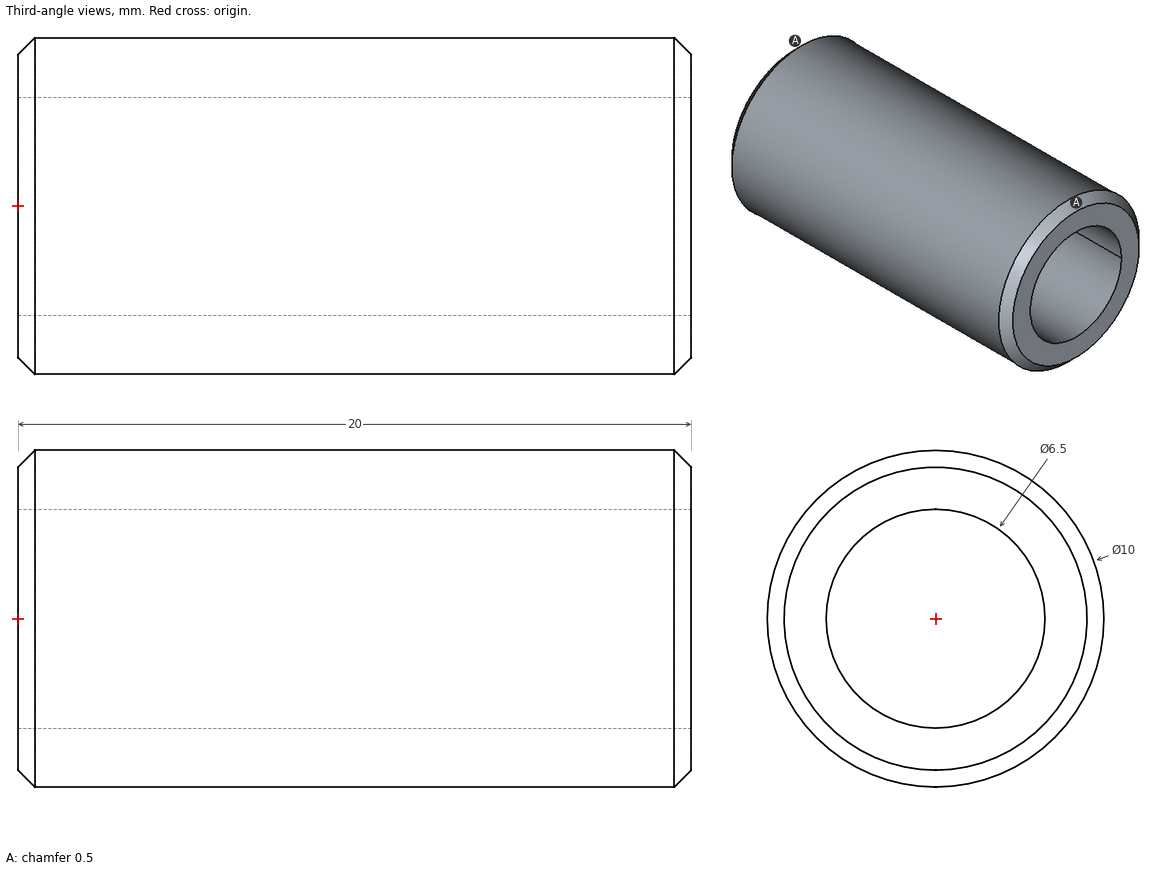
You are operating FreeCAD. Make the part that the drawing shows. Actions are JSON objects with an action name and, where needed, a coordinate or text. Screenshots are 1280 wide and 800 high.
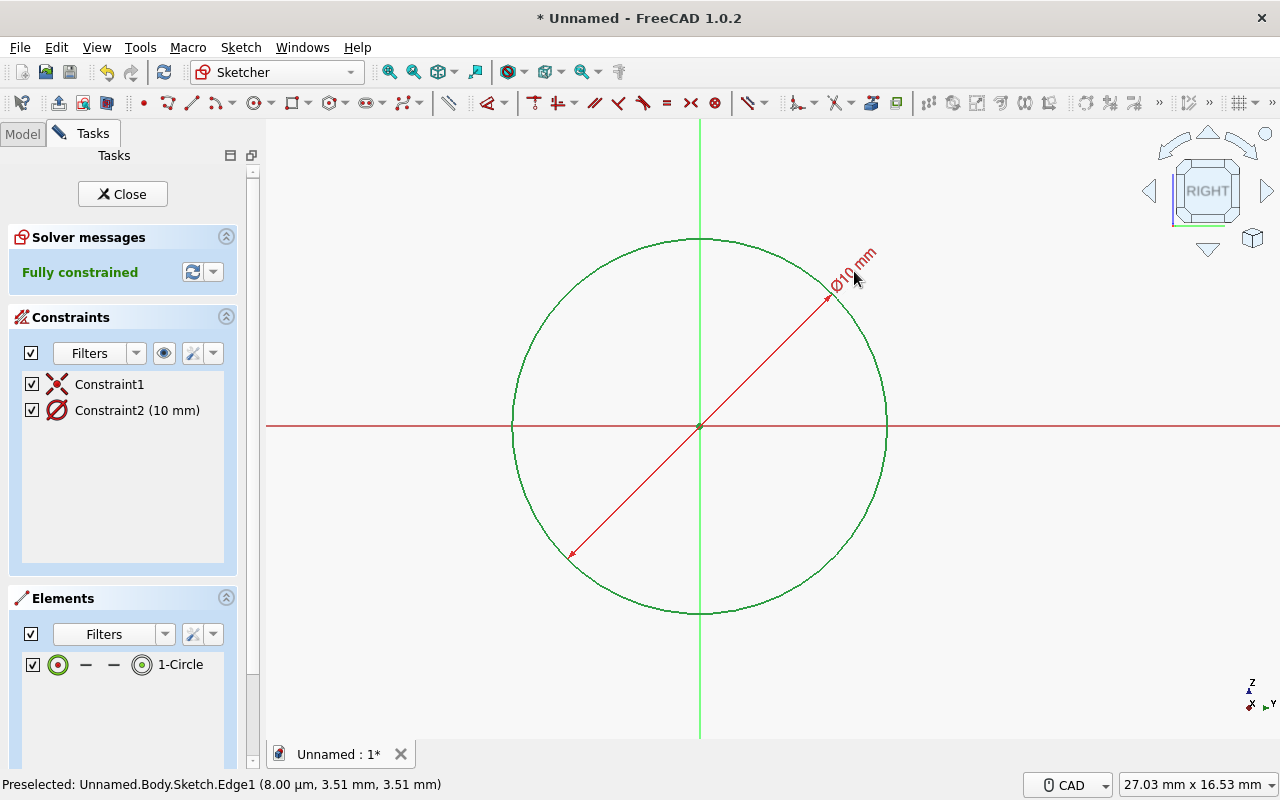
{"action": "left_click", "coordinate": [123, 194]}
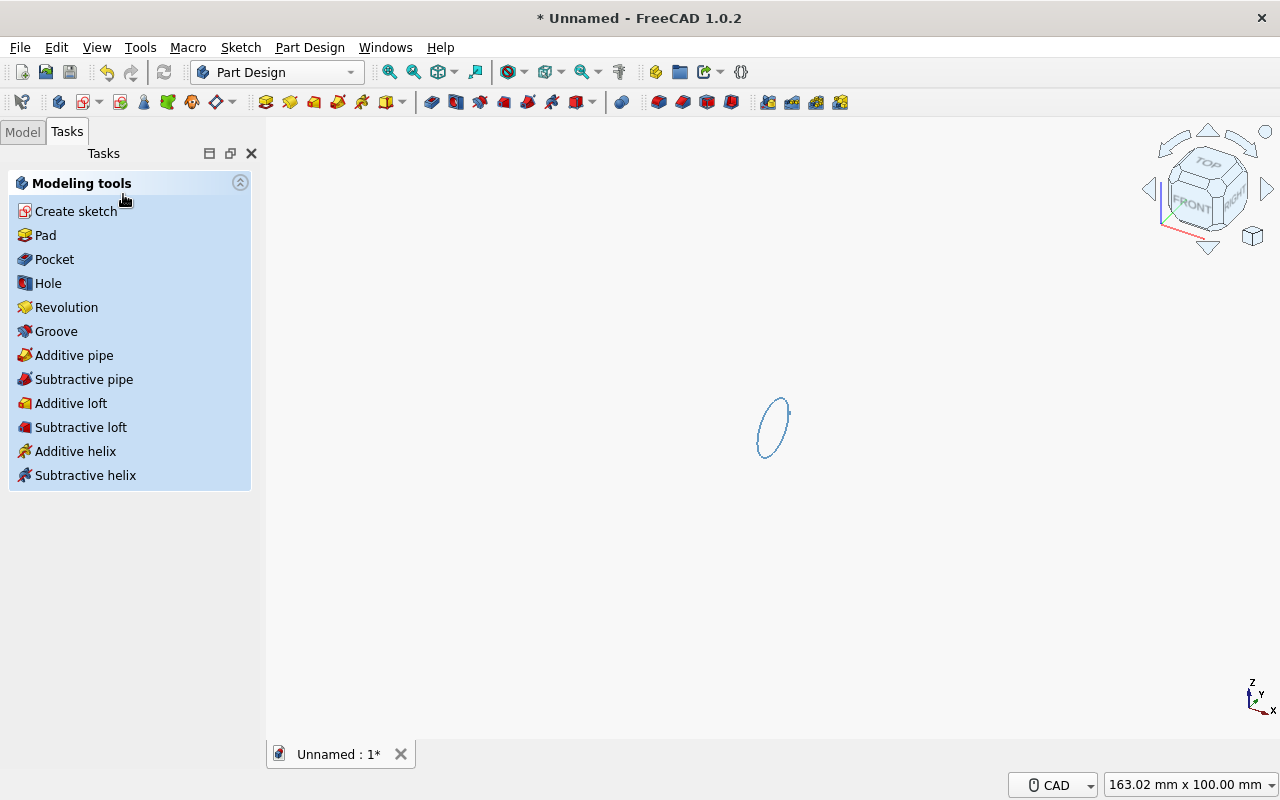
{"action": "left_click", "coordinate": [266, 102]}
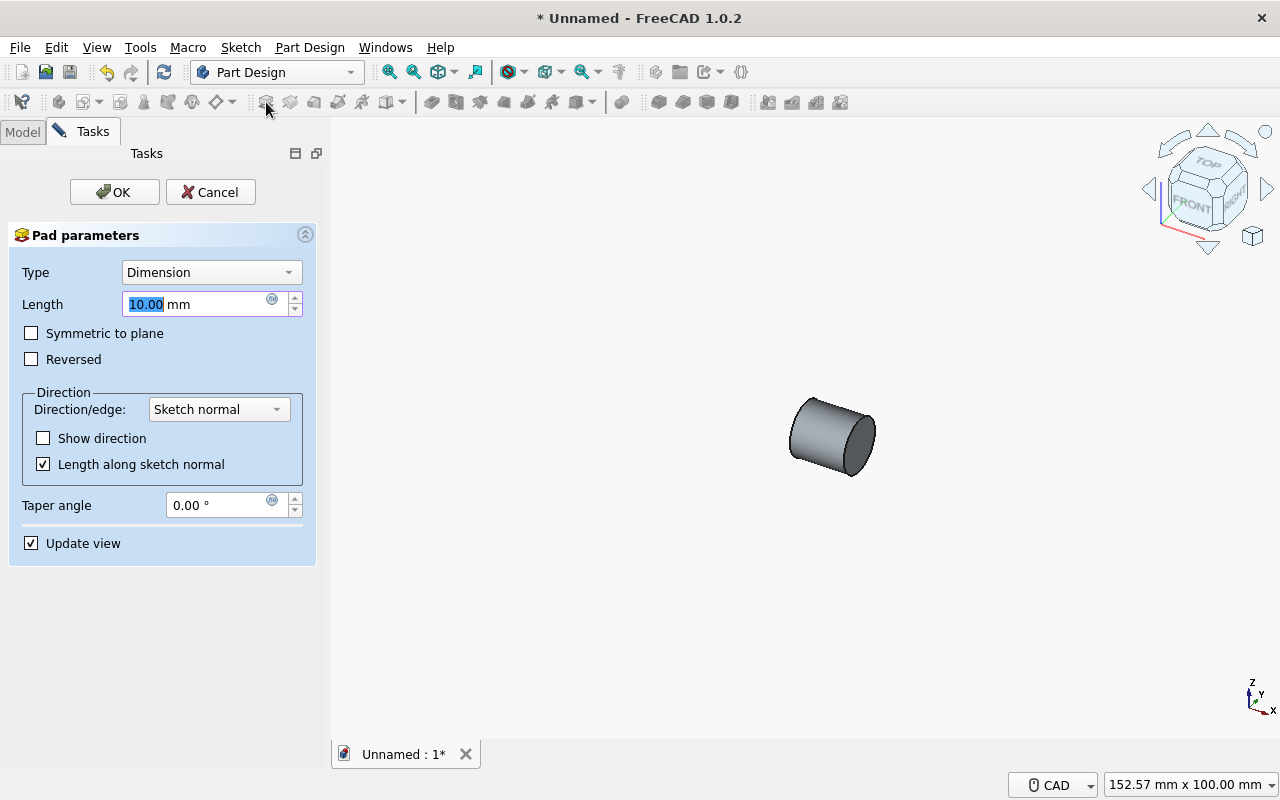
{"action": "type", "text": "20"}
{"action": "key", "text": "Tab"}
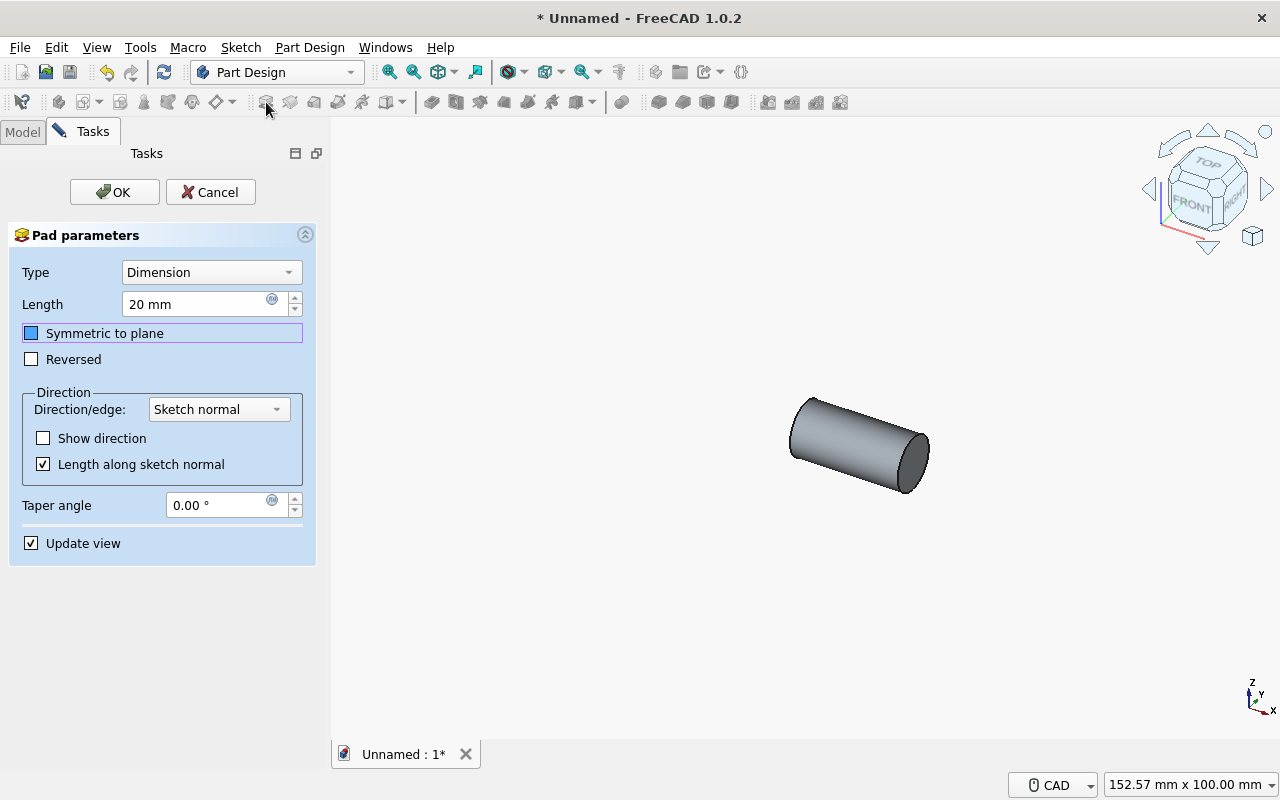
{"action": "left_click", "coordinate": [115, 192]}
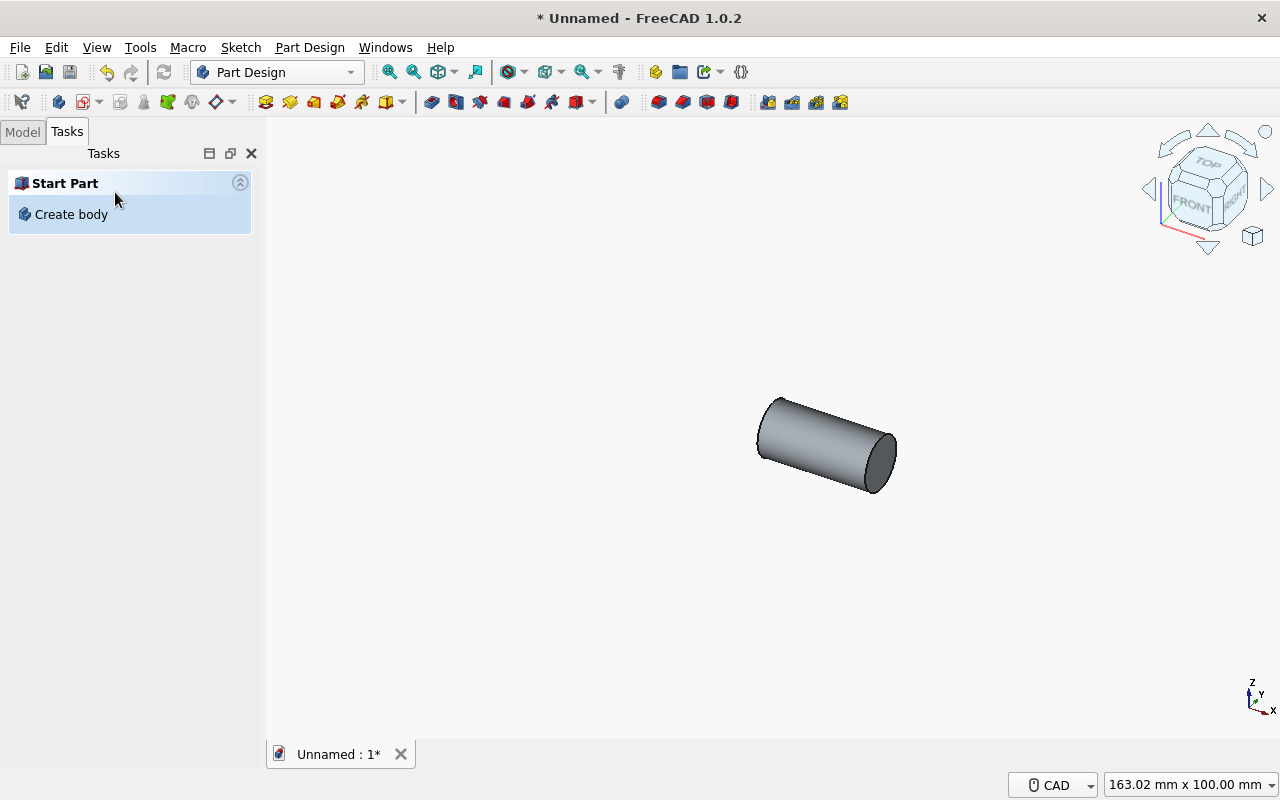
{"action": "left_click", "coordinate": [390, 72]}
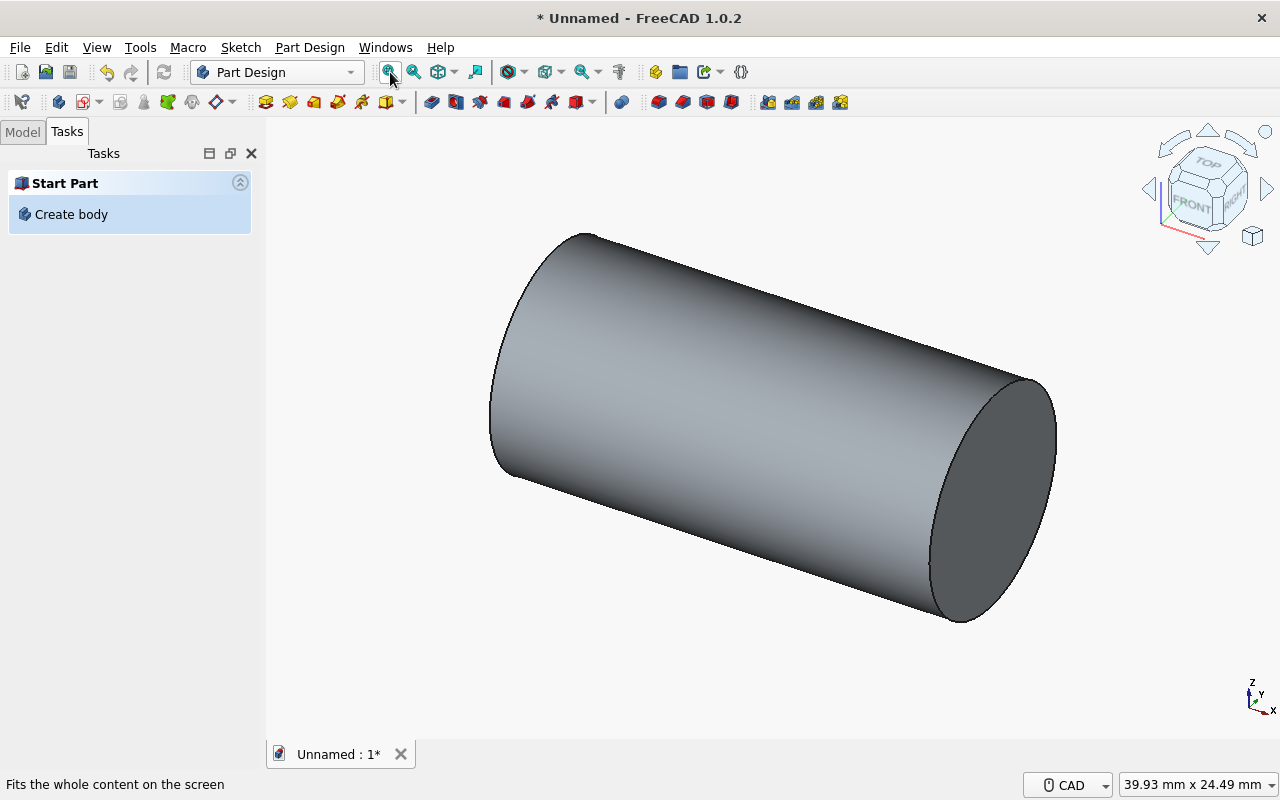
{"action": "left_click", "coordinate": [929, 563]}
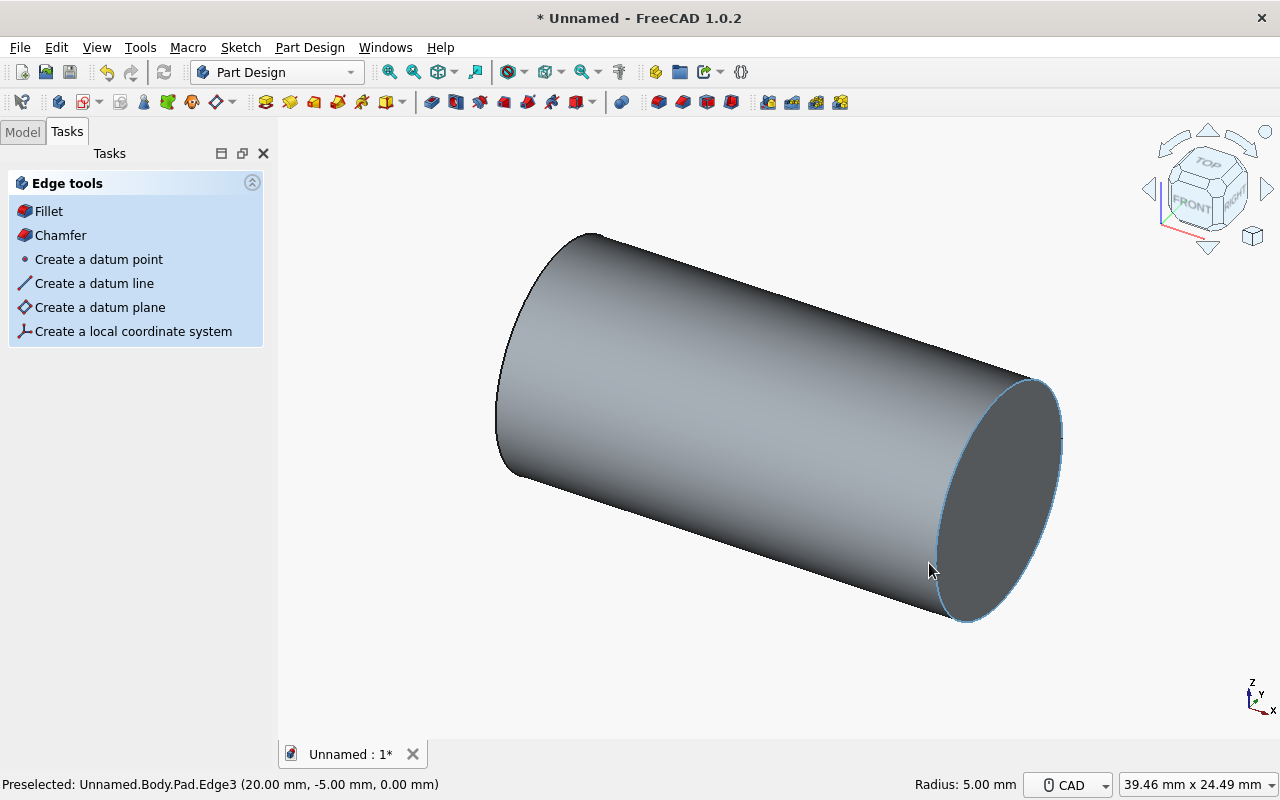
{"action": "key", "text": "0"}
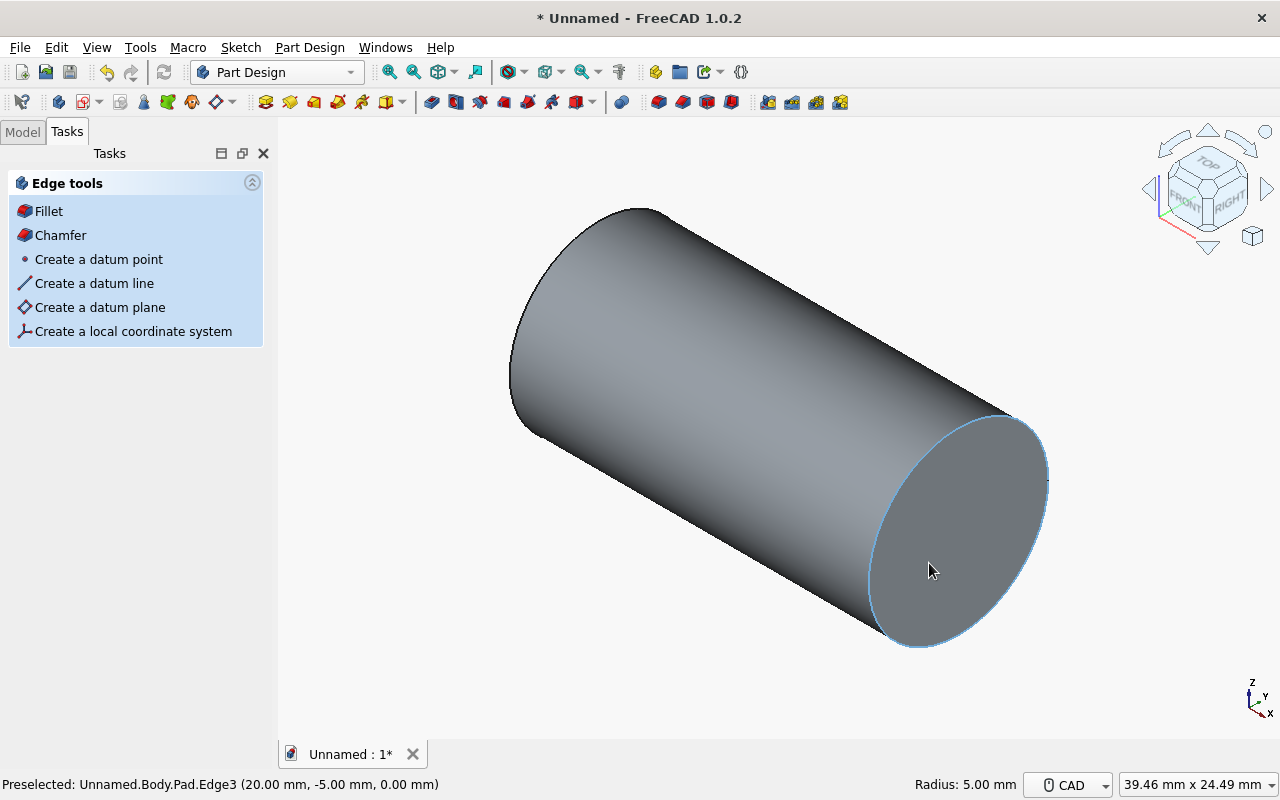
{"action": "key", "text": "2"}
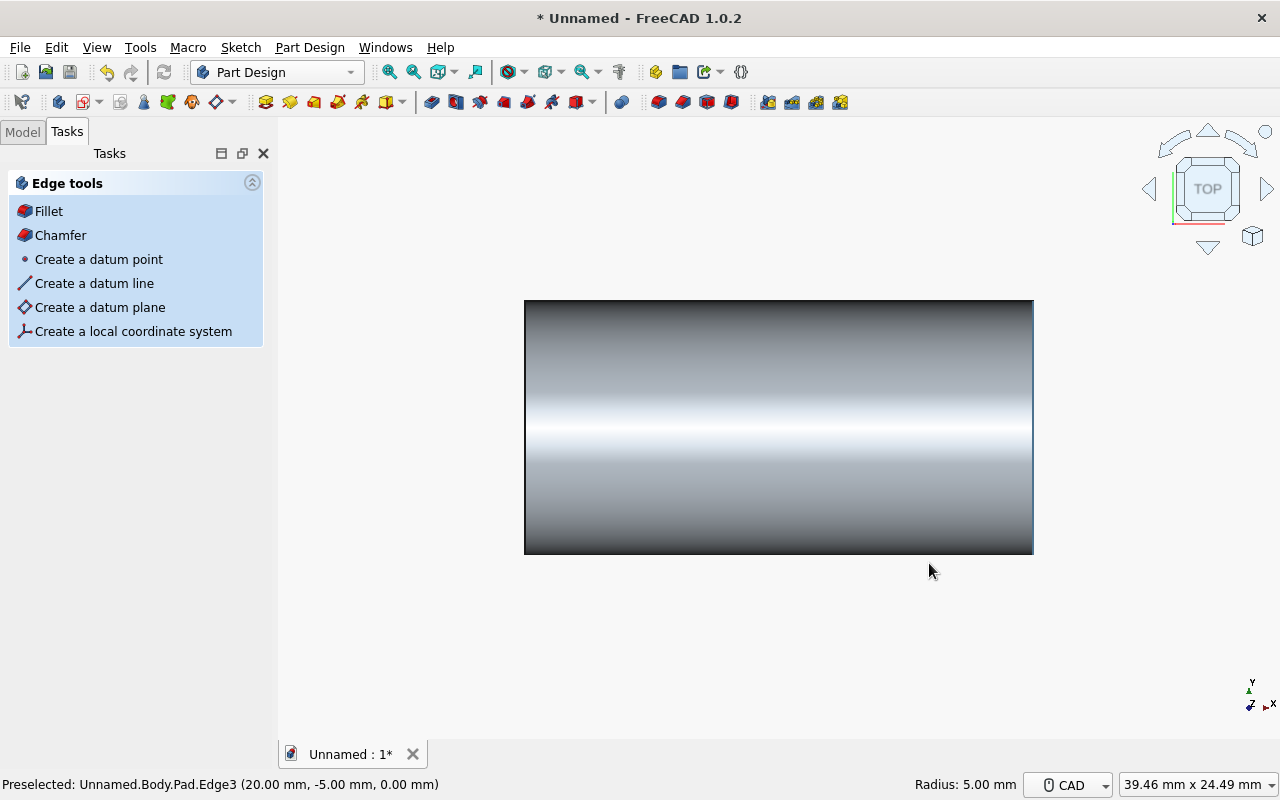
{"action": "left_click", "coordinate": [525, 530], "text": "ctrl"}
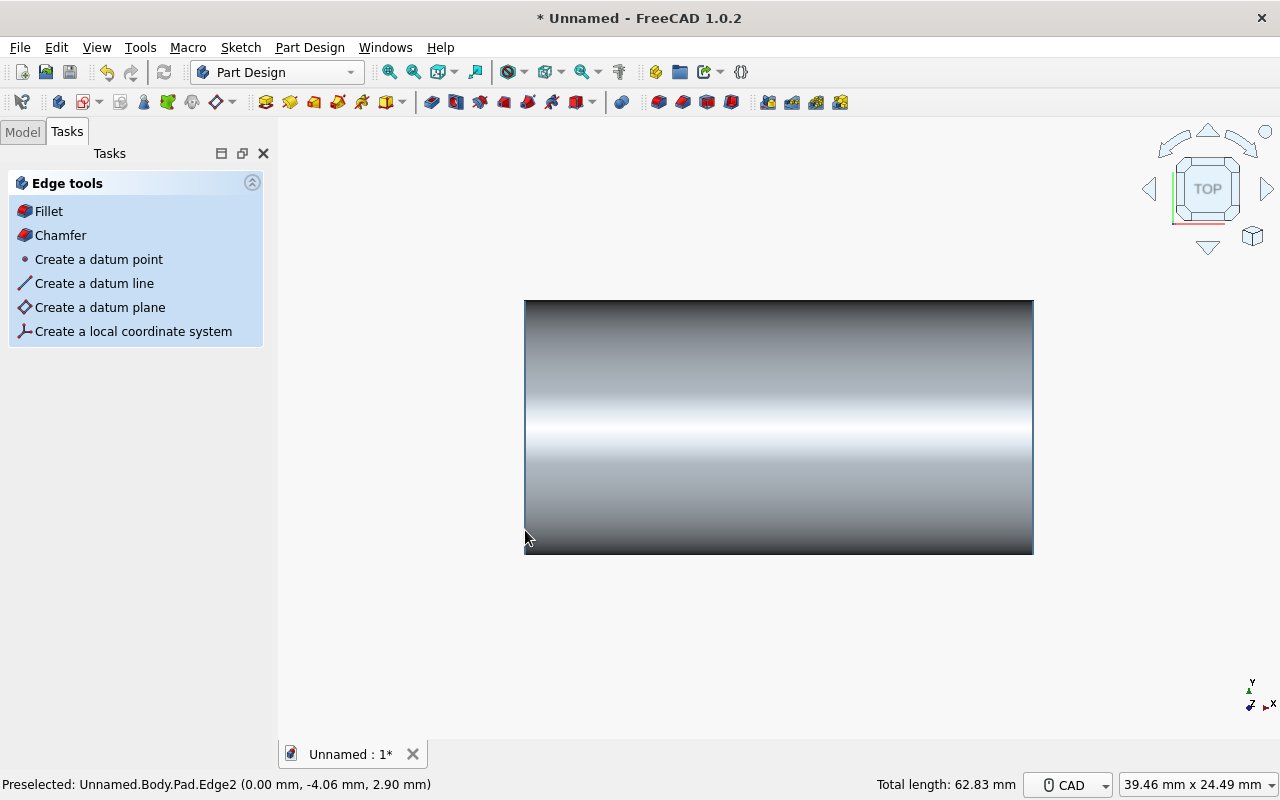
{"action": "left_click", "coordinate": [684, 102]}